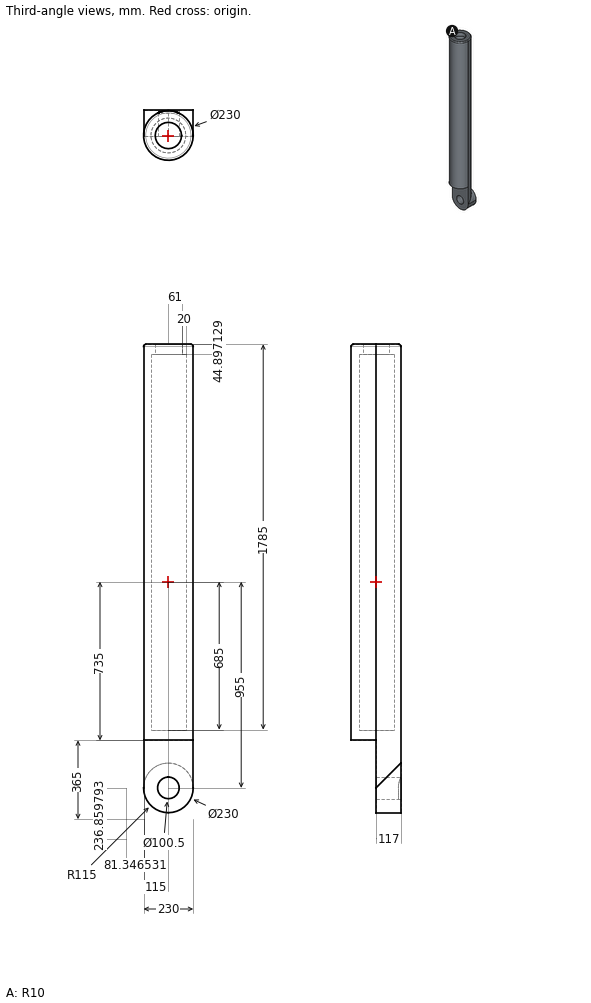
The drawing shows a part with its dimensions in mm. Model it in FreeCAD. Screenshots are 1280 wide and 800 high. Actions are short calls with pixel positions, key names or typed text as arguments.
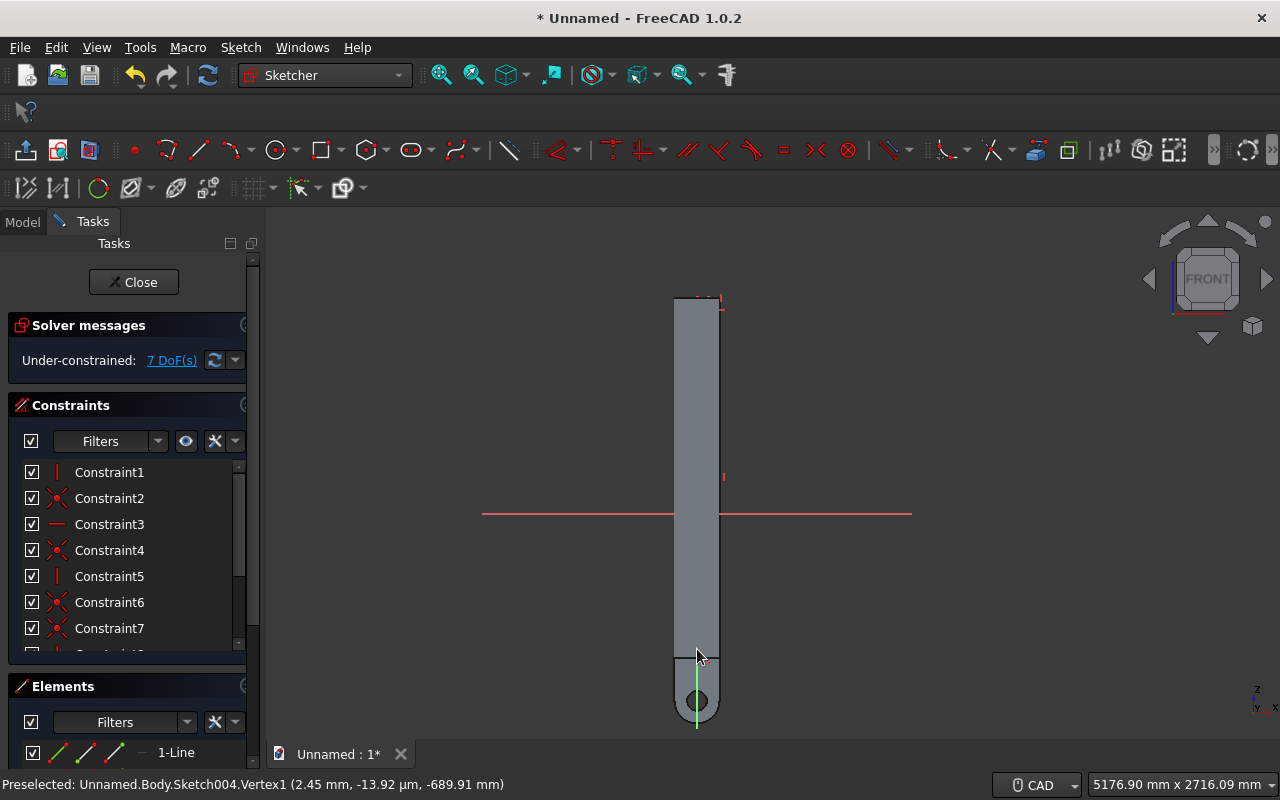
scroll(711, 308, up, 10)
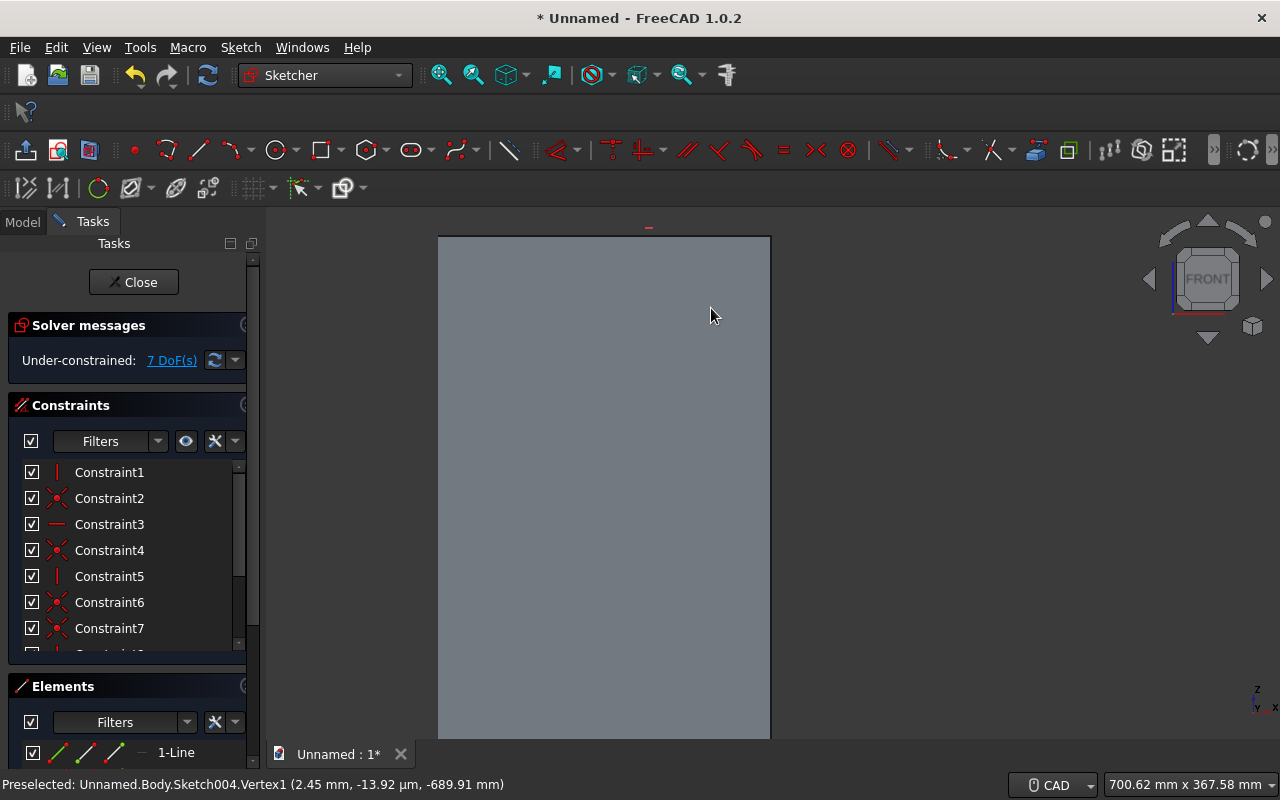
click(706, 307)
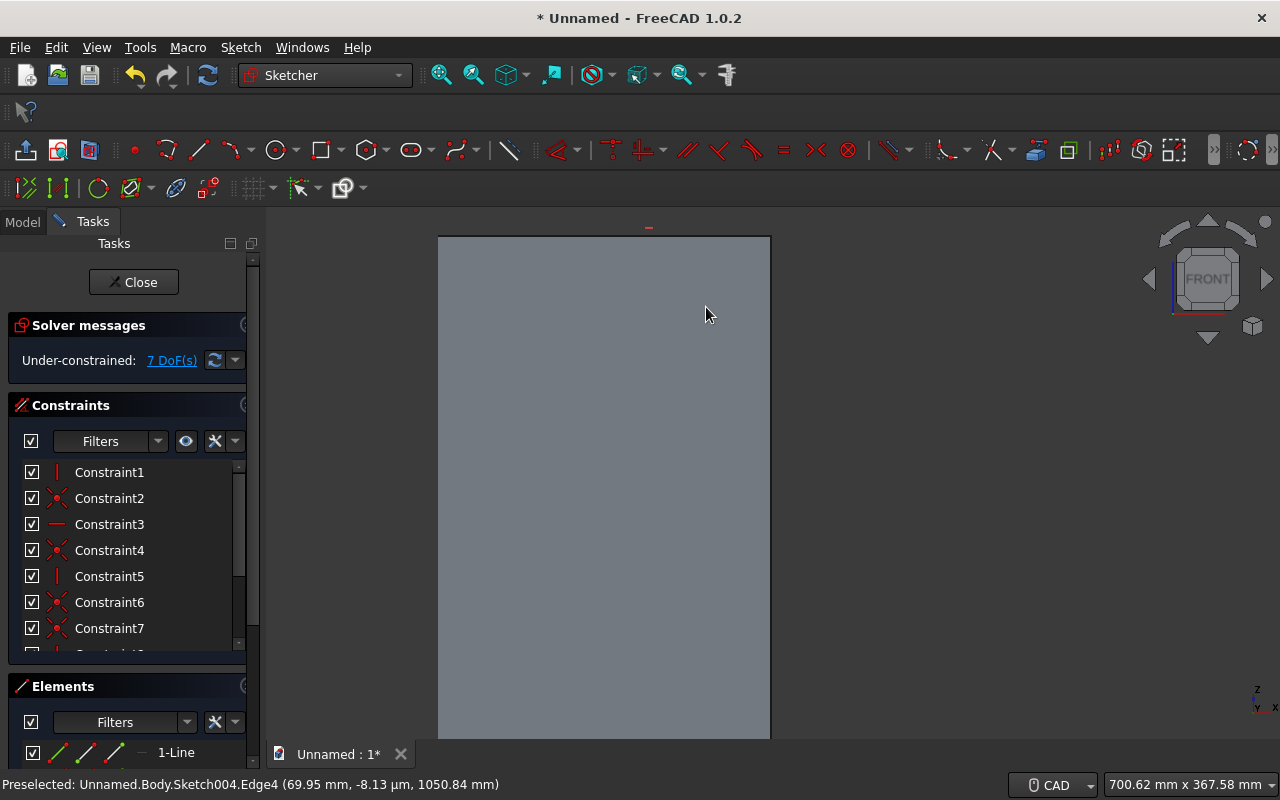
key(h)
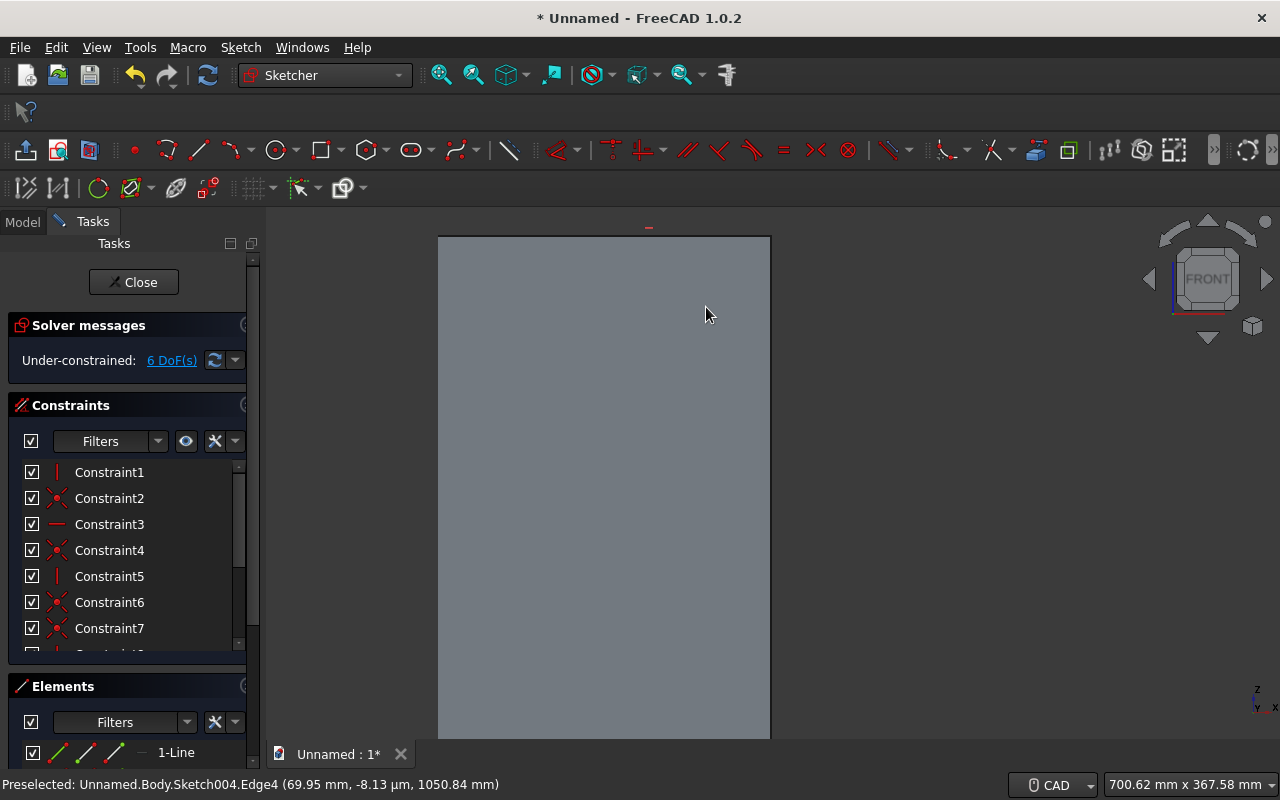
scroll(711, 308, down, 10)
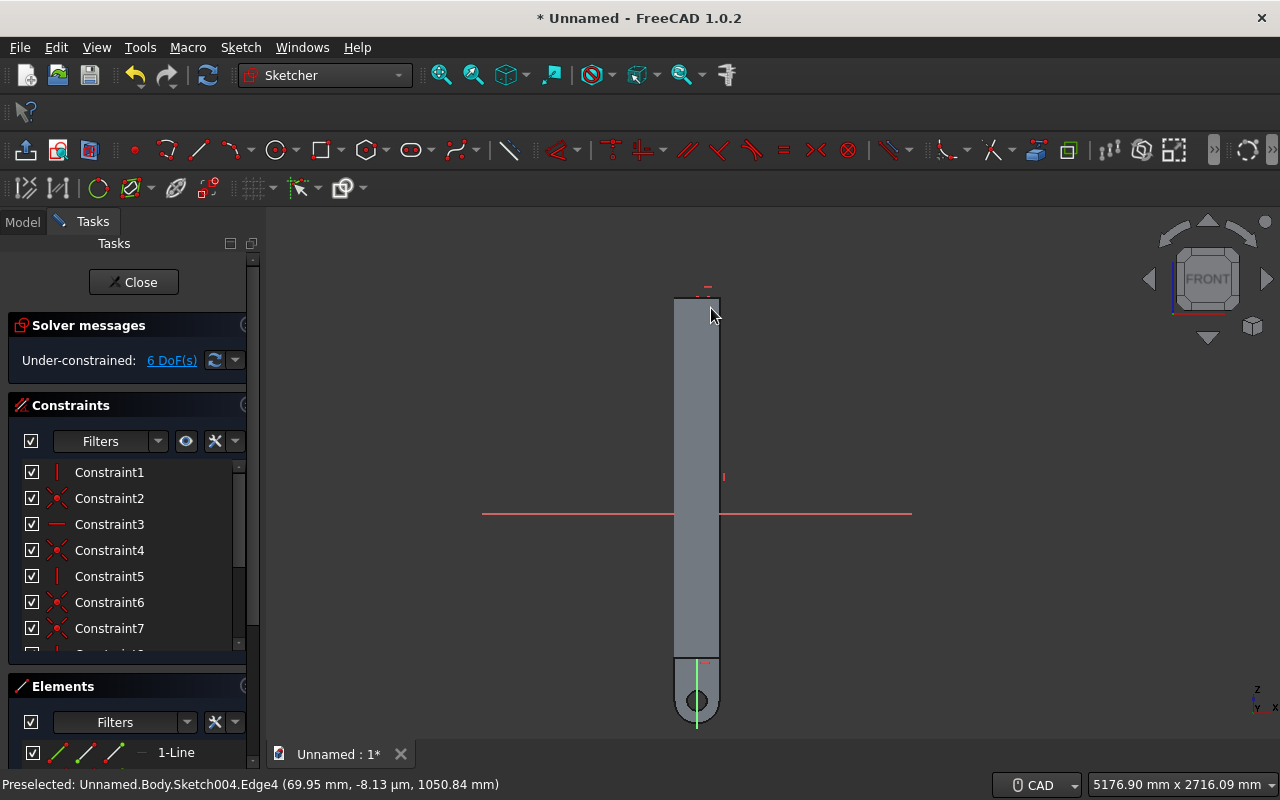
click(697, 649)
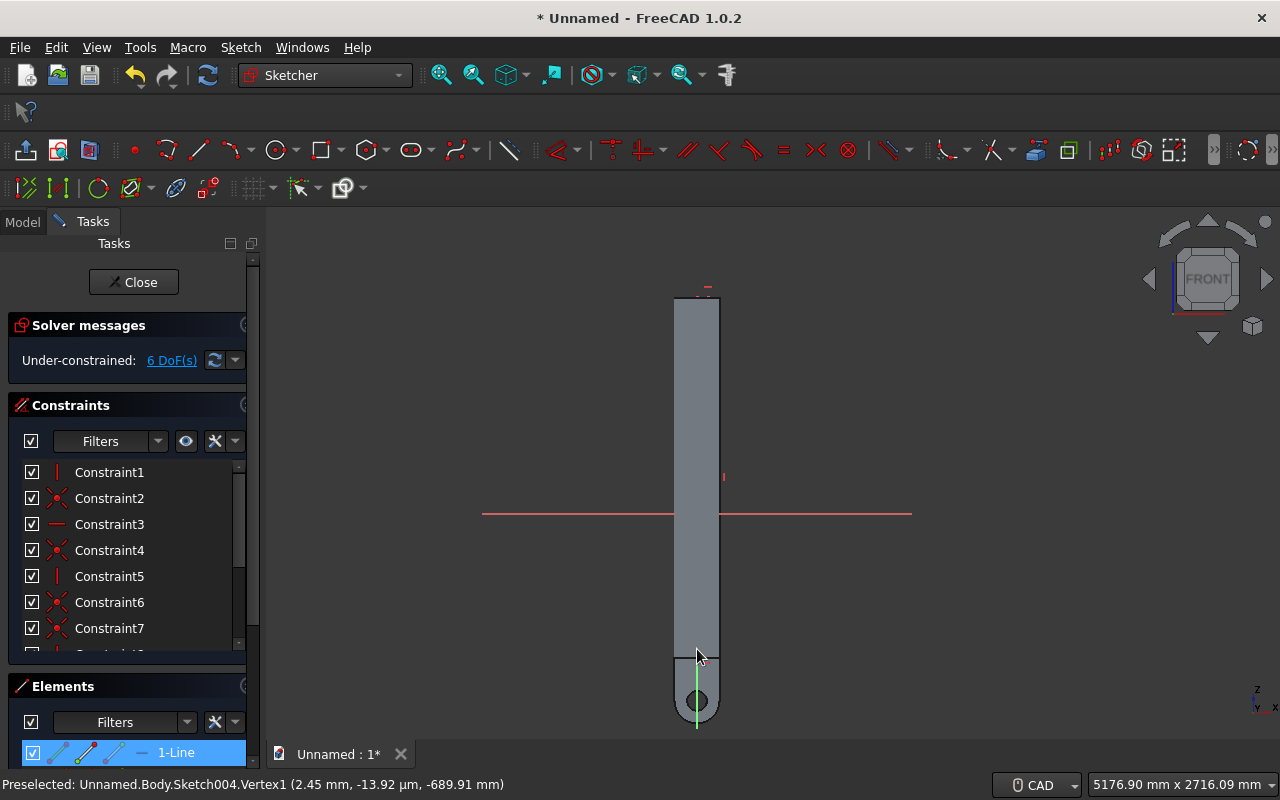
click(697, 677)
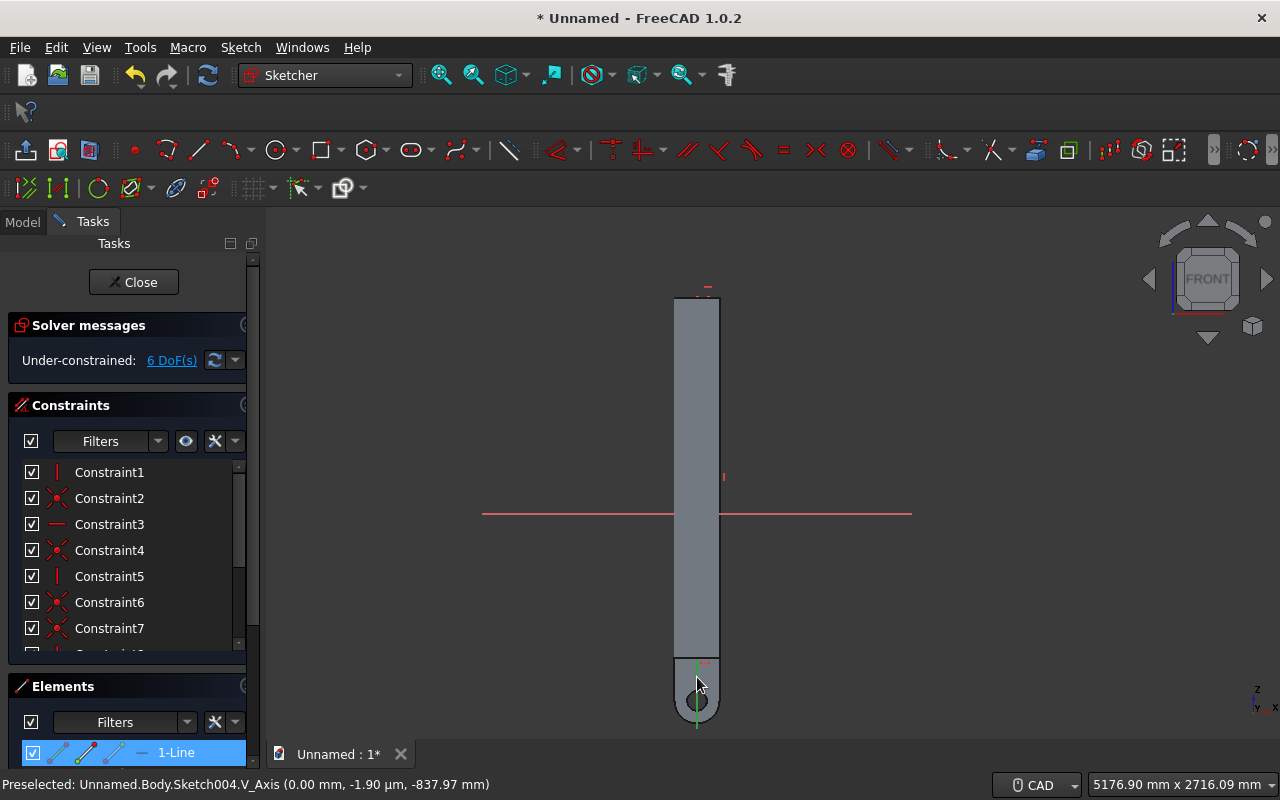
click(612, 150)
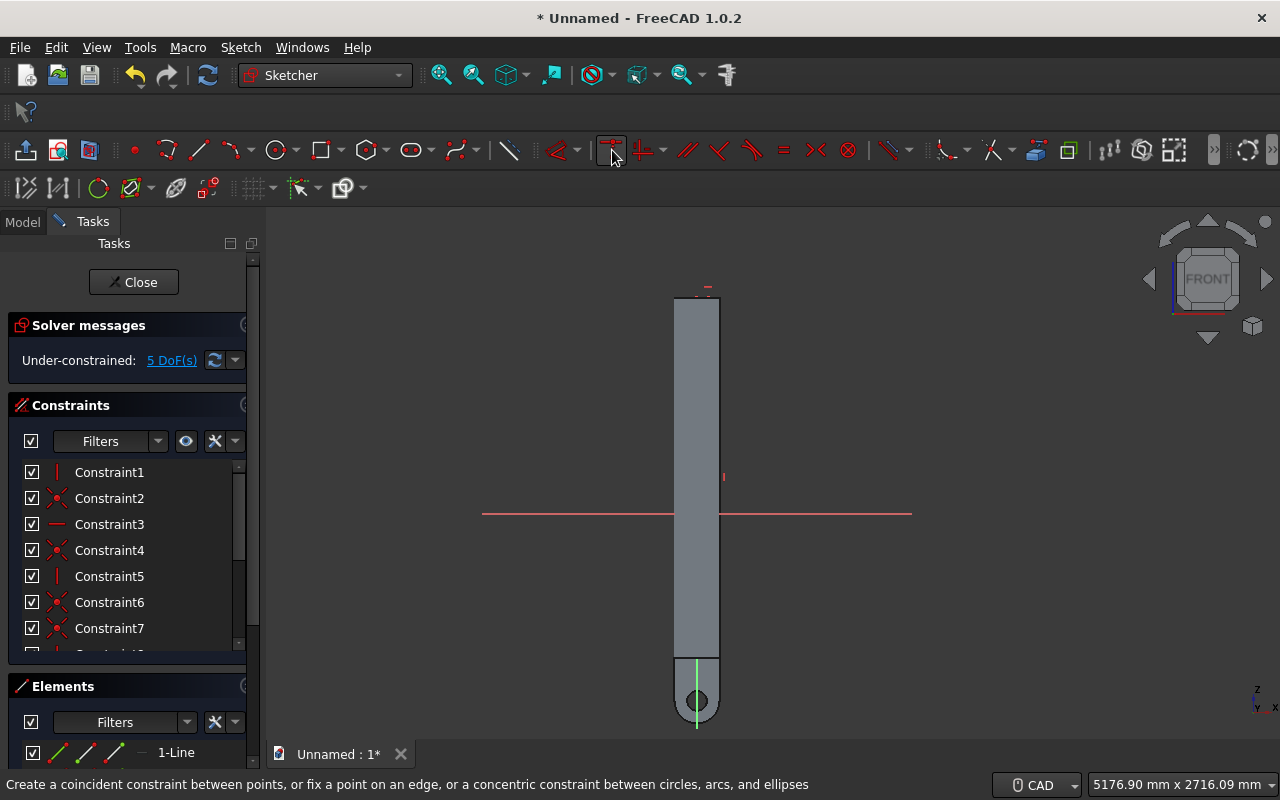
key(d)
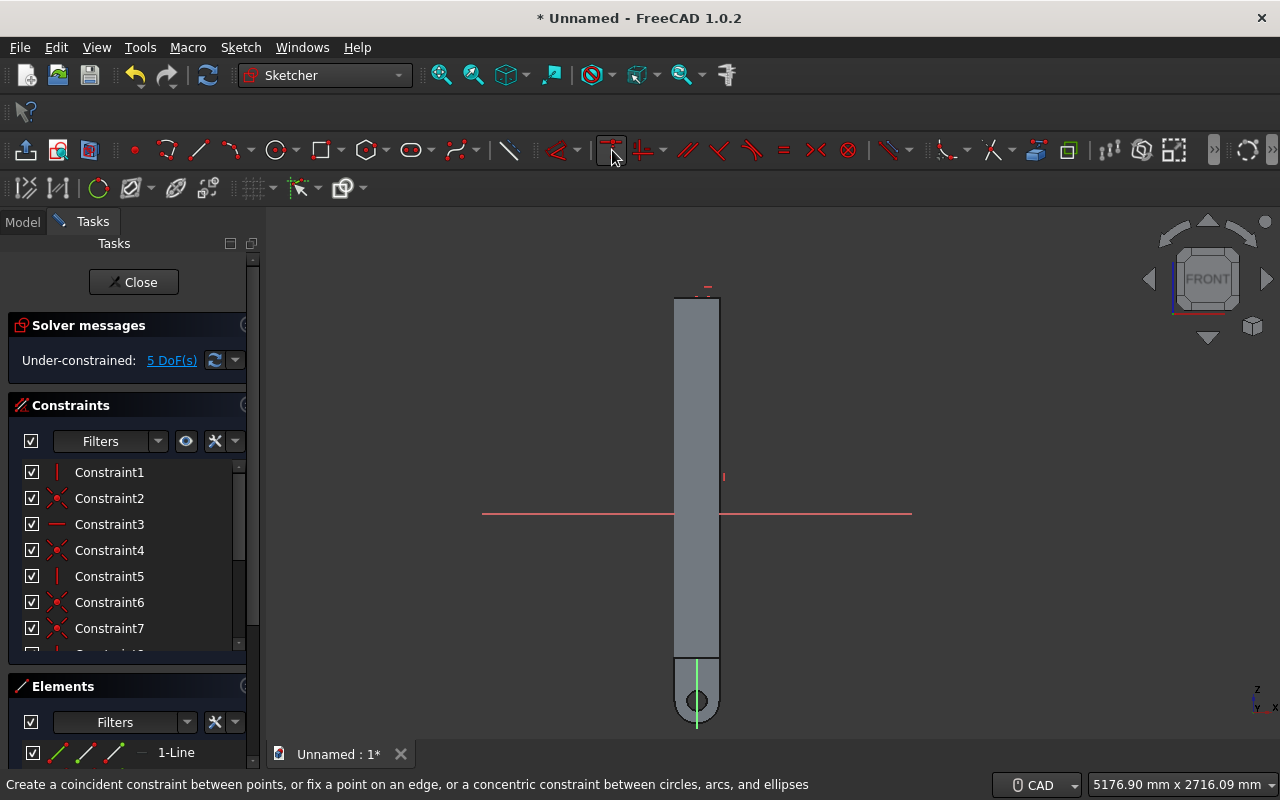
scroll(703, 299, up, 7)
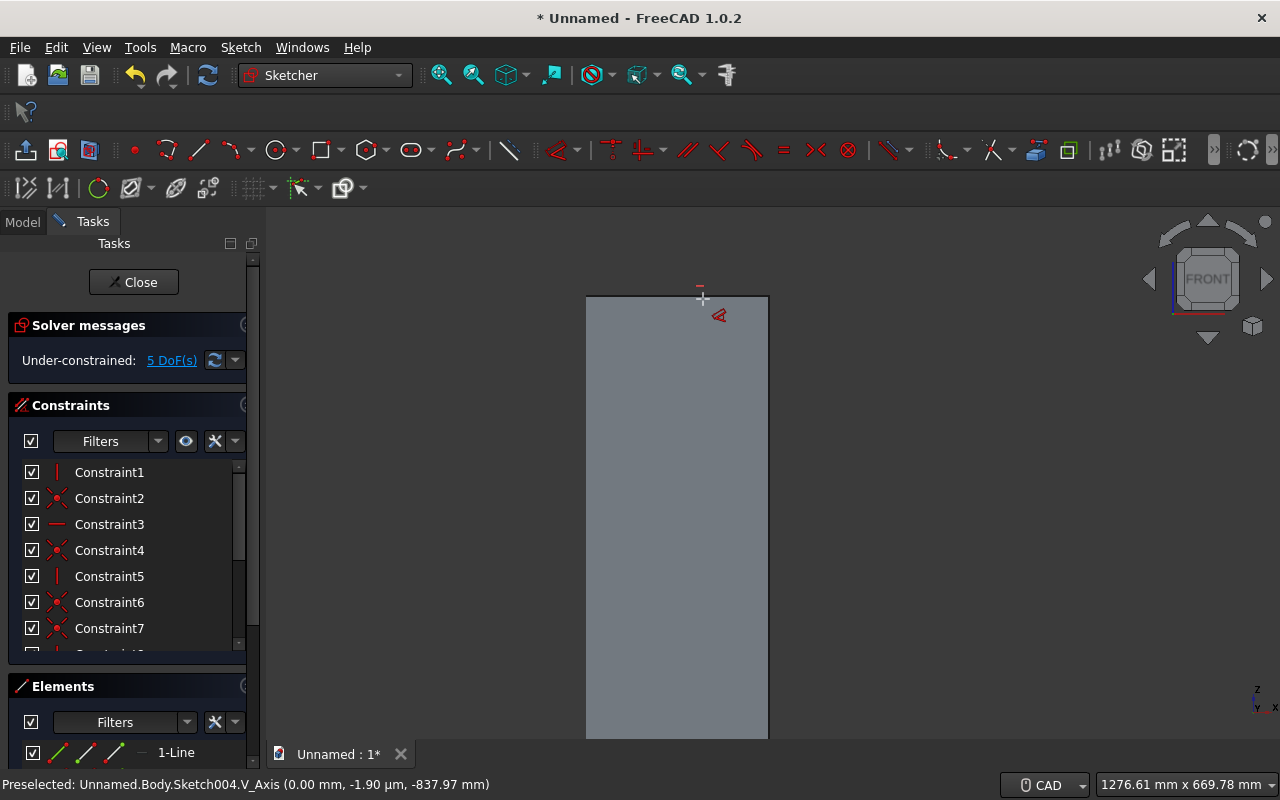
click(701, 299)
click(701, 265)